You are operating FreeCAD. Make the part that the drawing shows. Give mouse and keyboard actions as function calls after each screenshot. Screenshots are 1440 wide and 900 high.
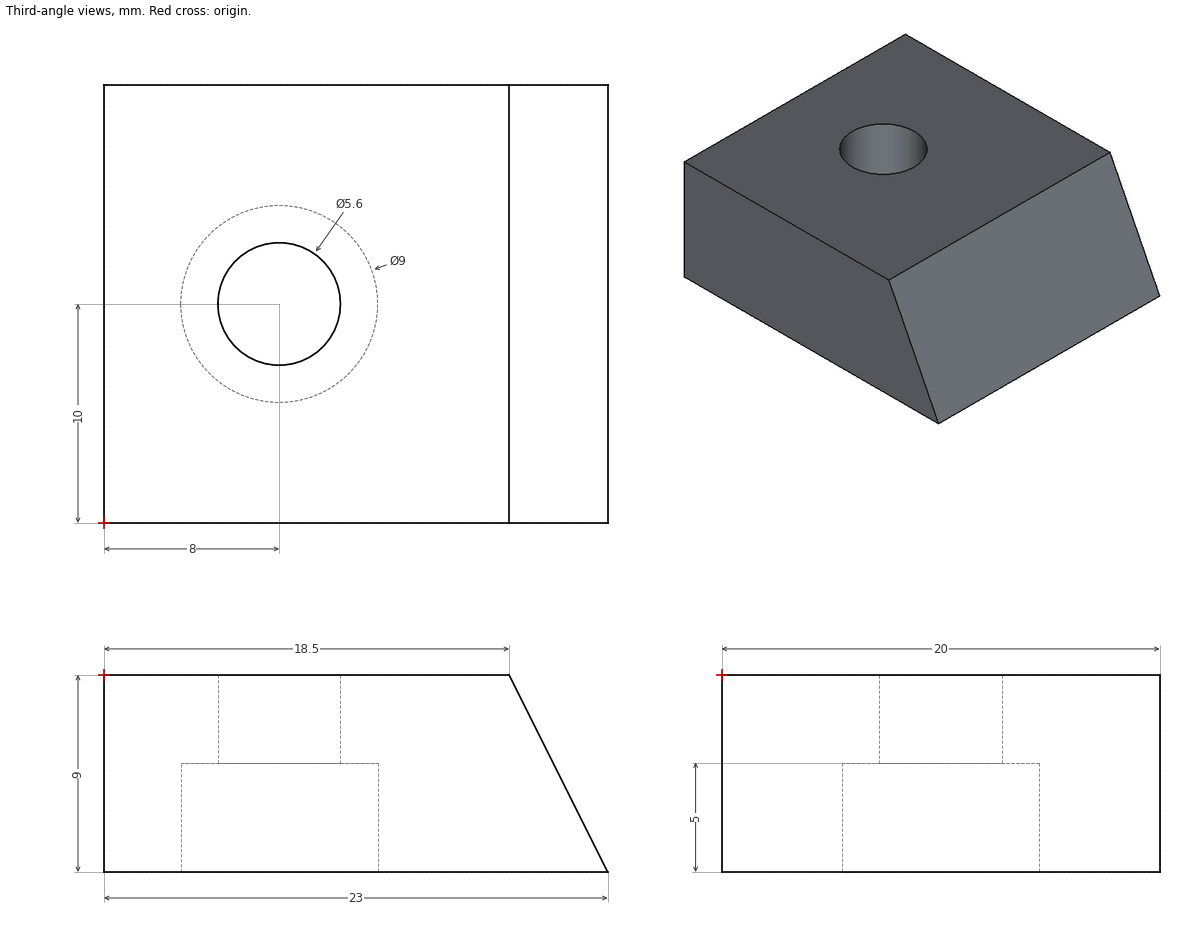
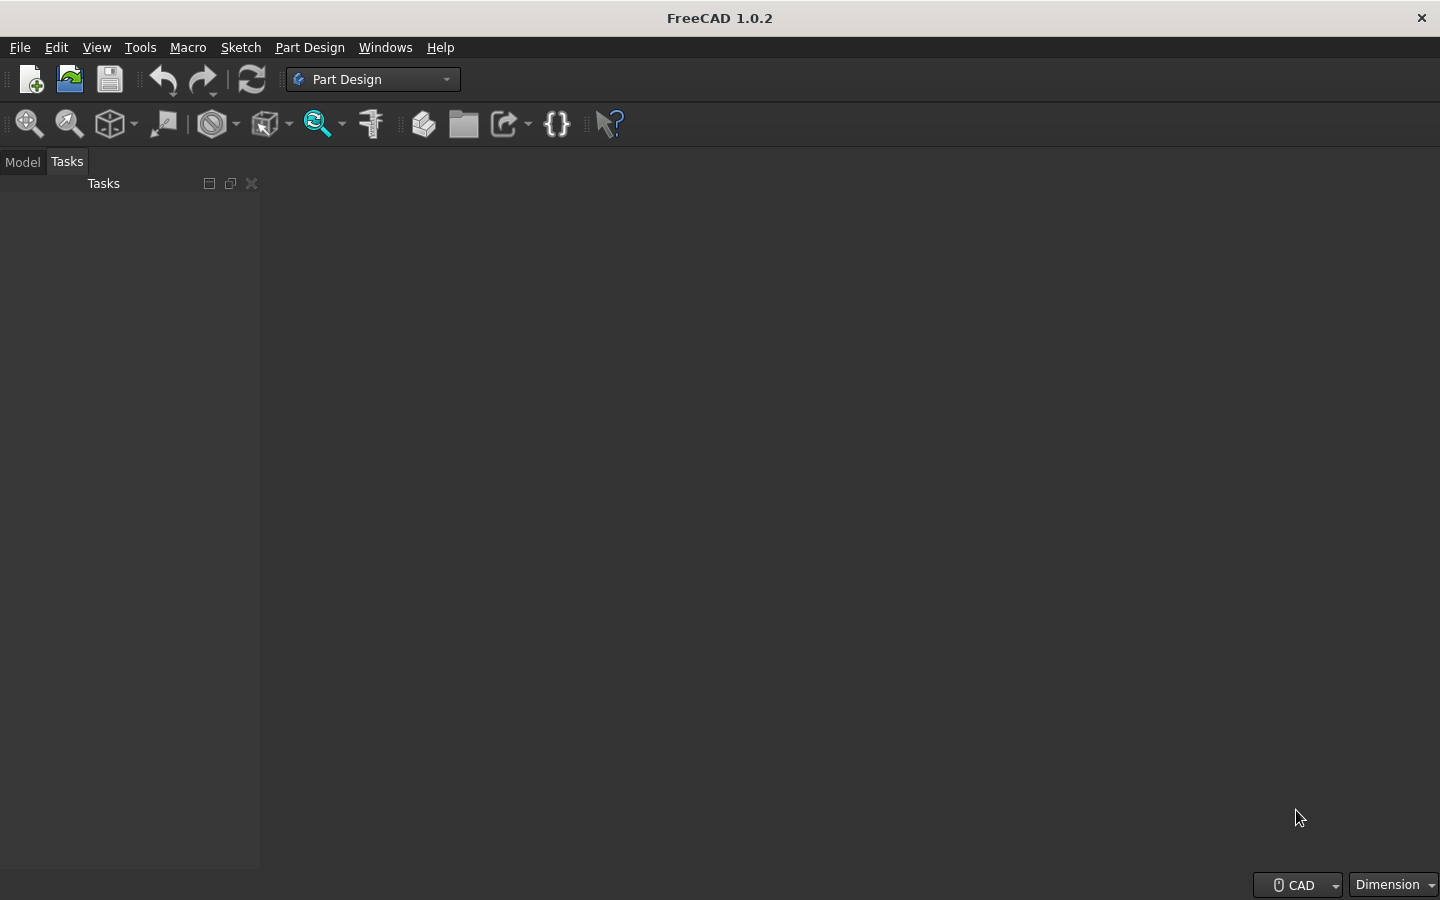
click(30, 80)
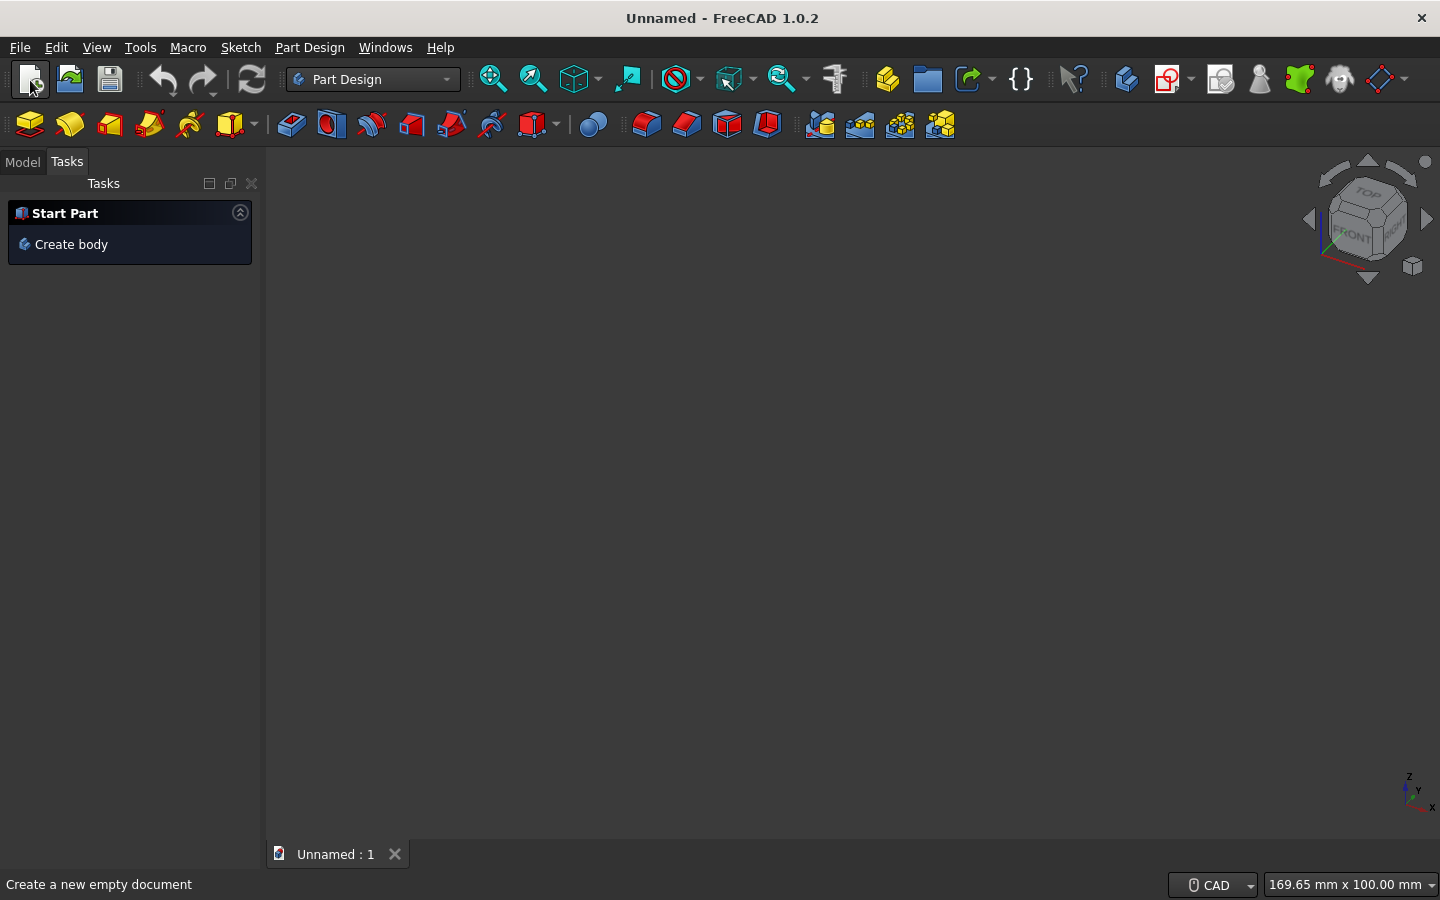
click(1168, 80)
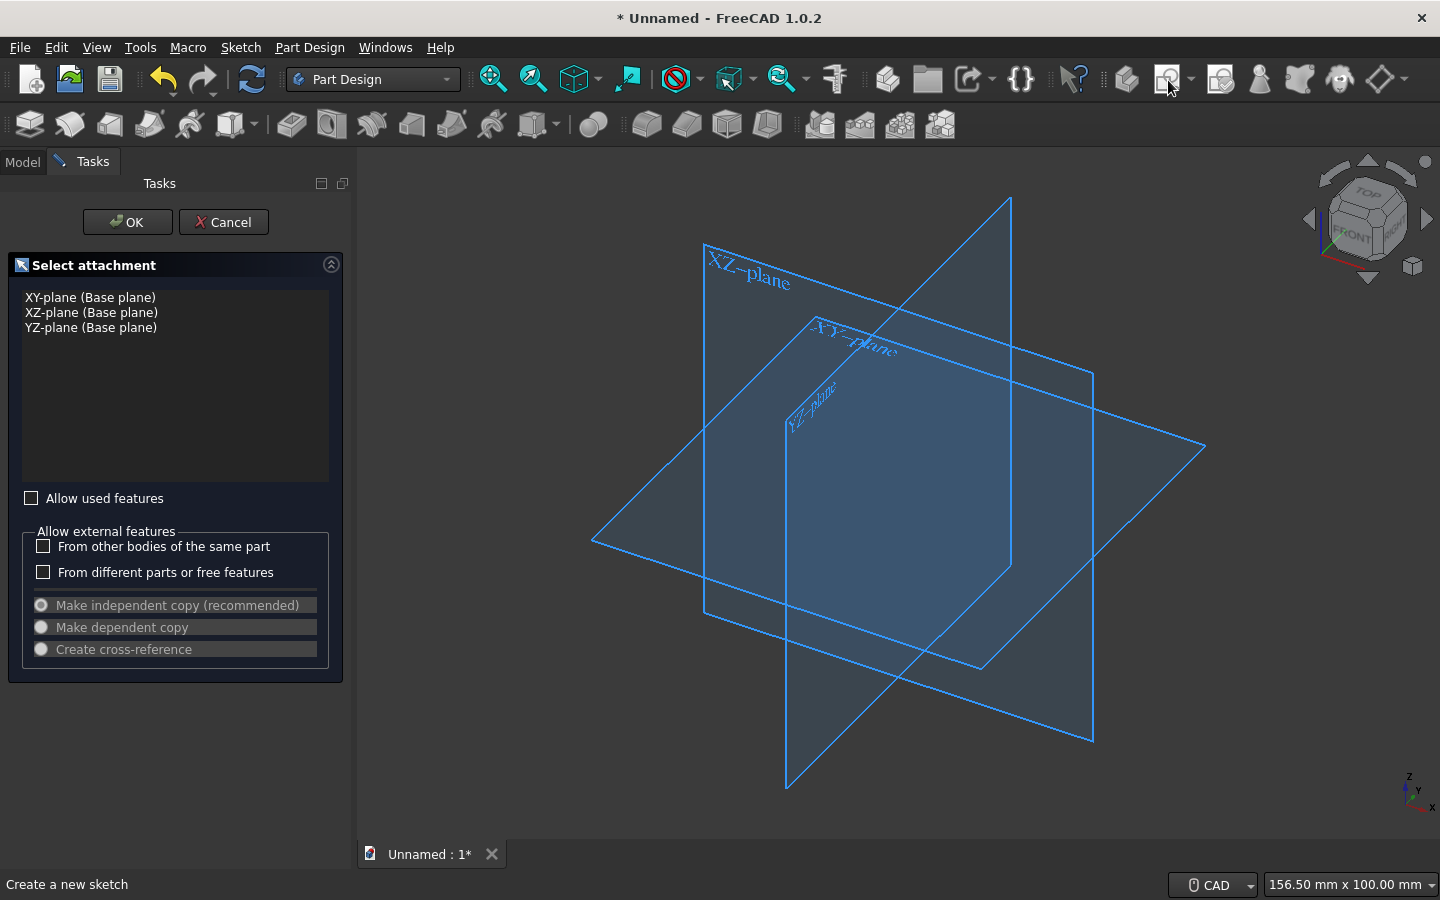
click(82, 312)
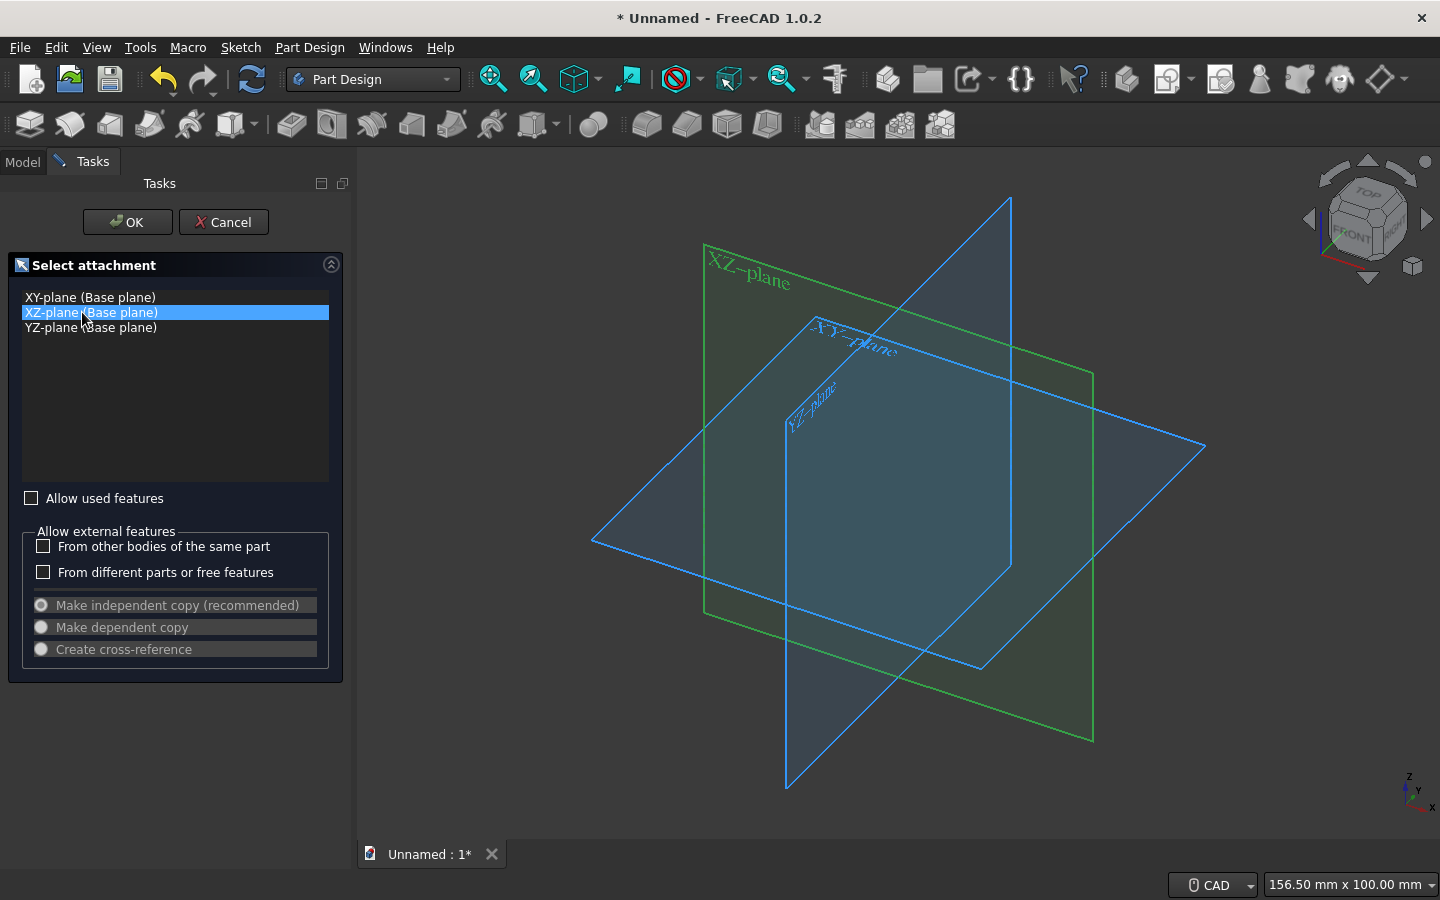
click(128, 222)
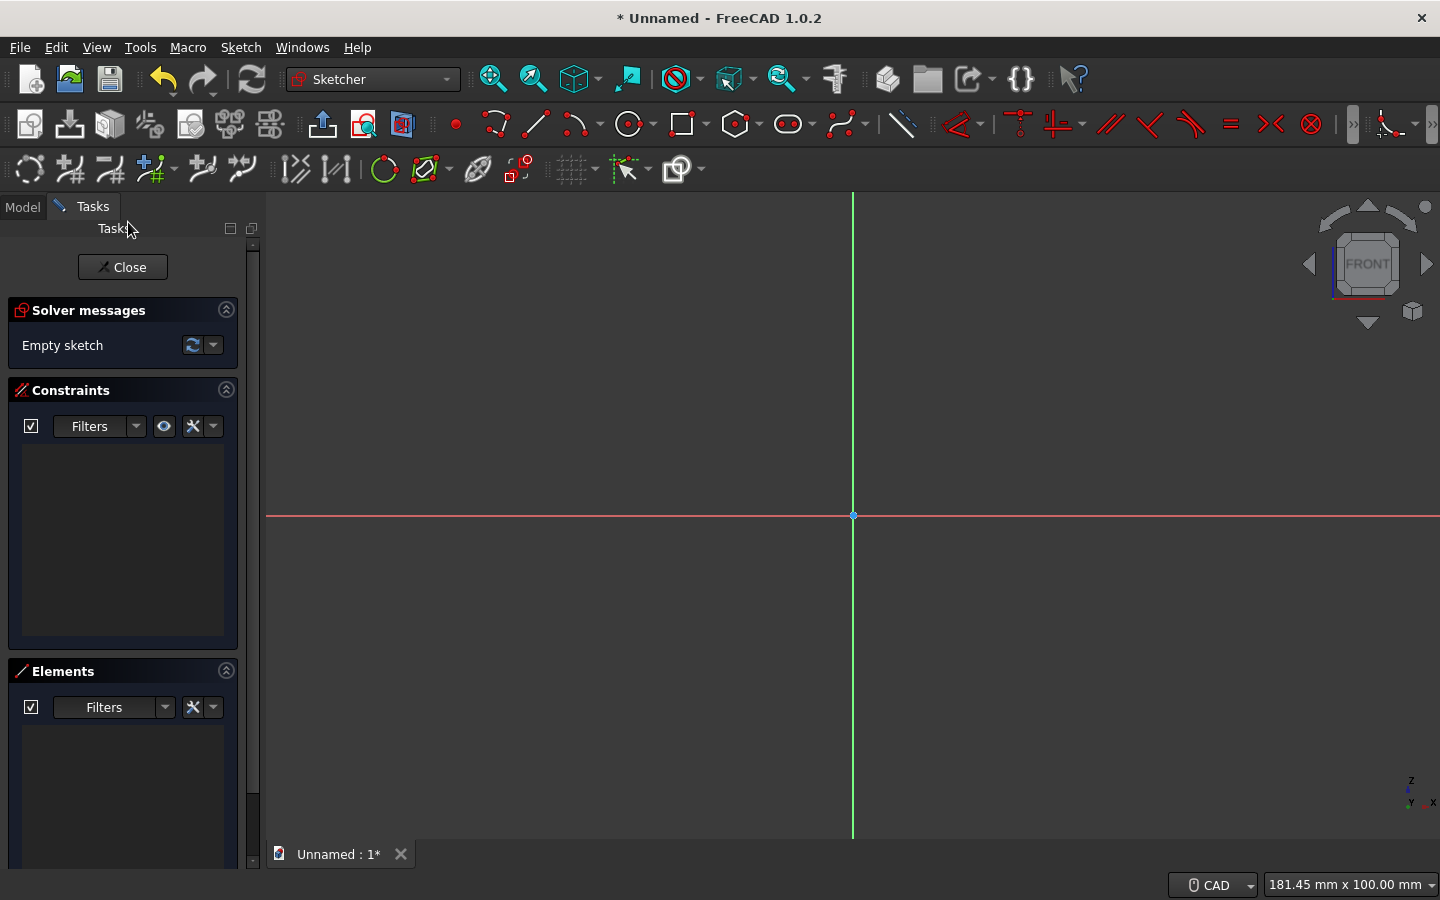
scroll(964, 552, up, 8)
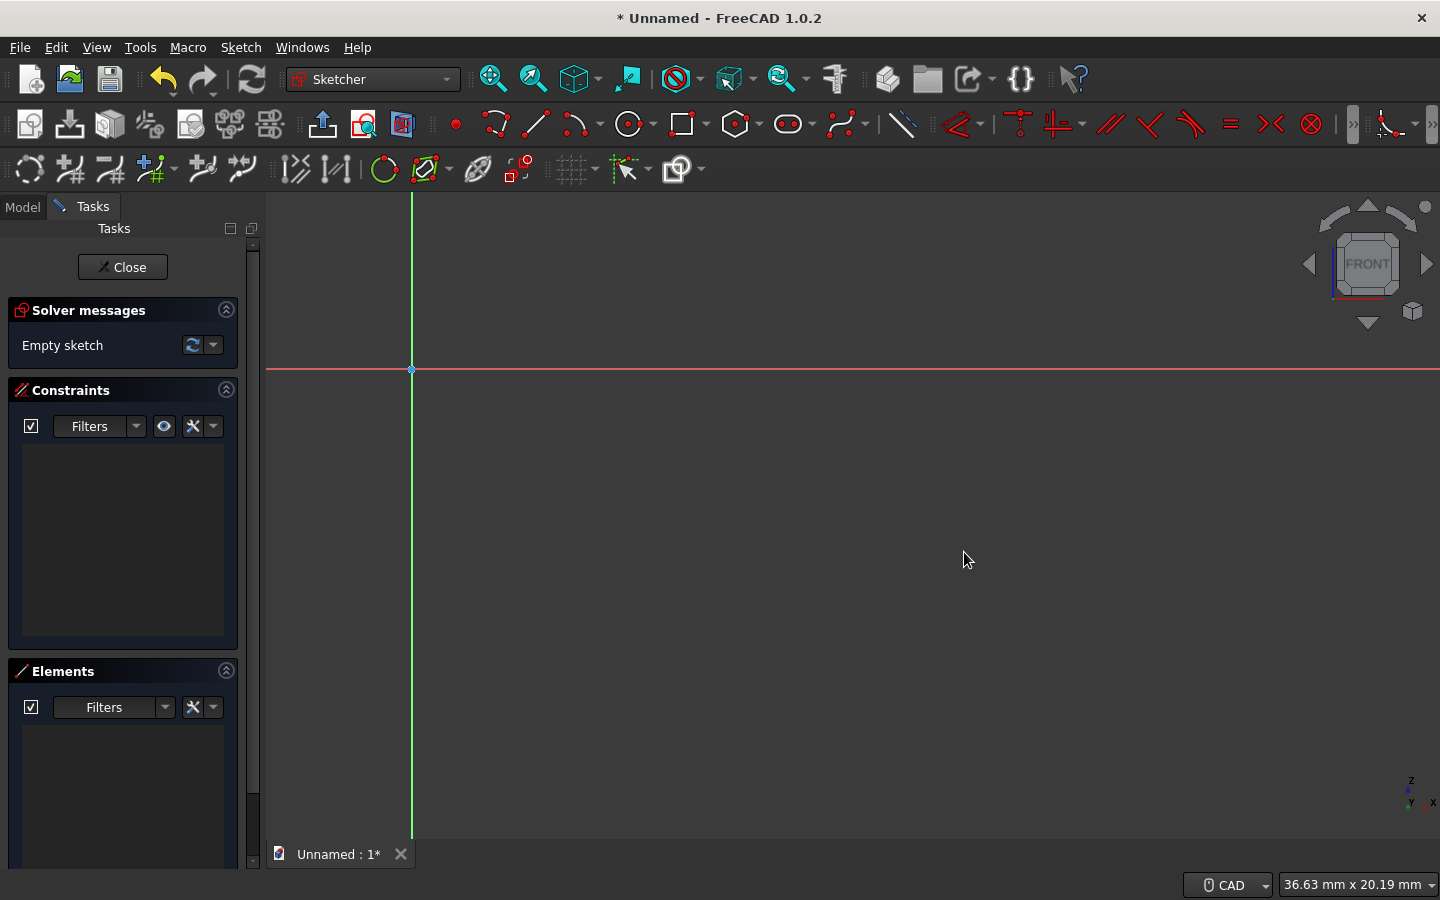
click(496, 124)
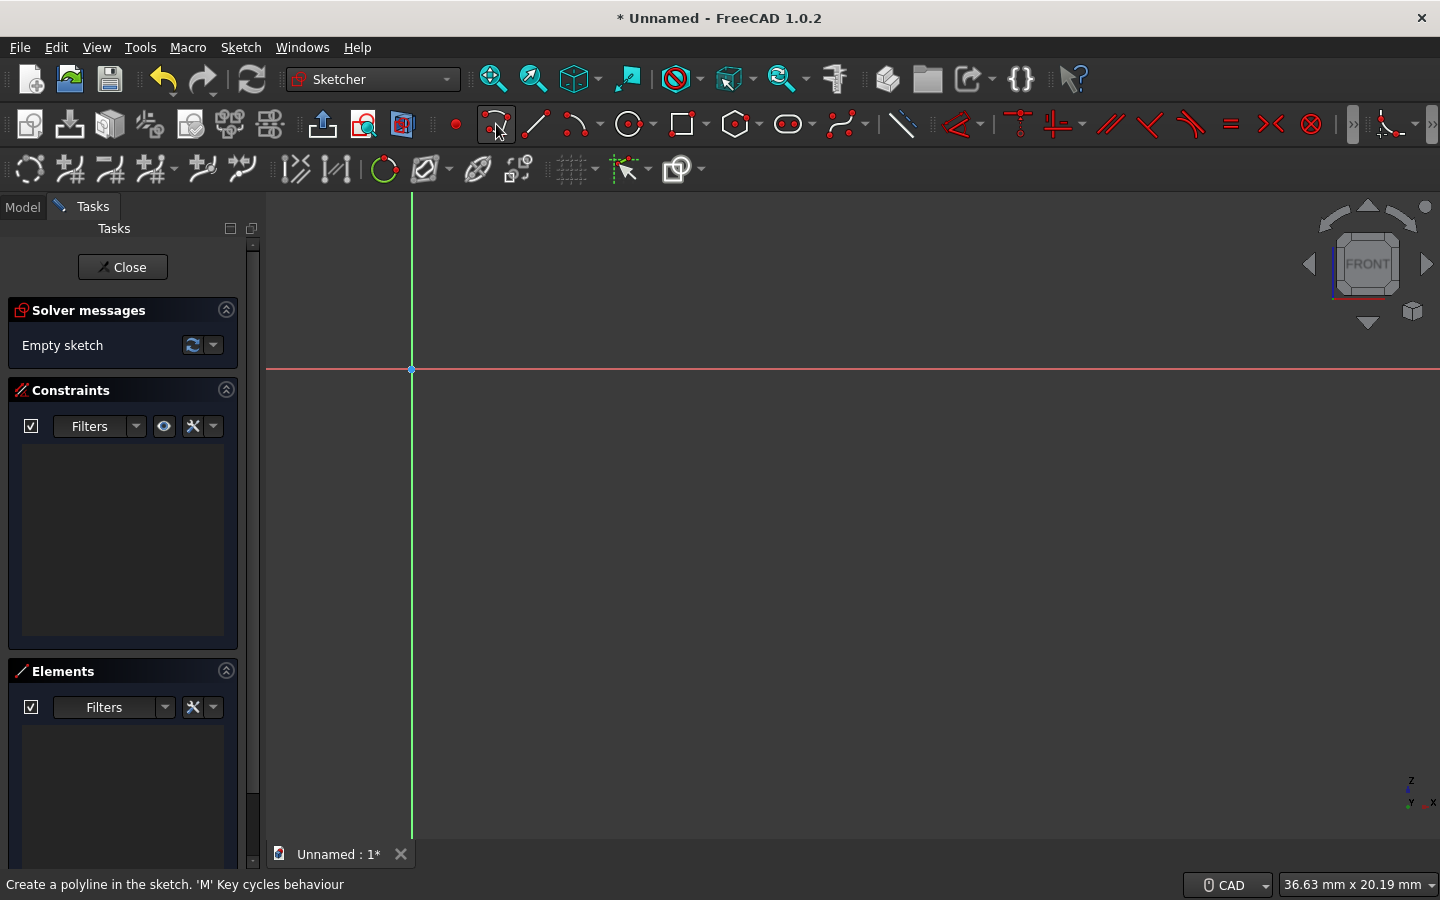
click(412, 369)
click(1005, 378)
click(1149, 657)
click(421, 657)
click(412, 369)
key(Escape)
key(Escape)